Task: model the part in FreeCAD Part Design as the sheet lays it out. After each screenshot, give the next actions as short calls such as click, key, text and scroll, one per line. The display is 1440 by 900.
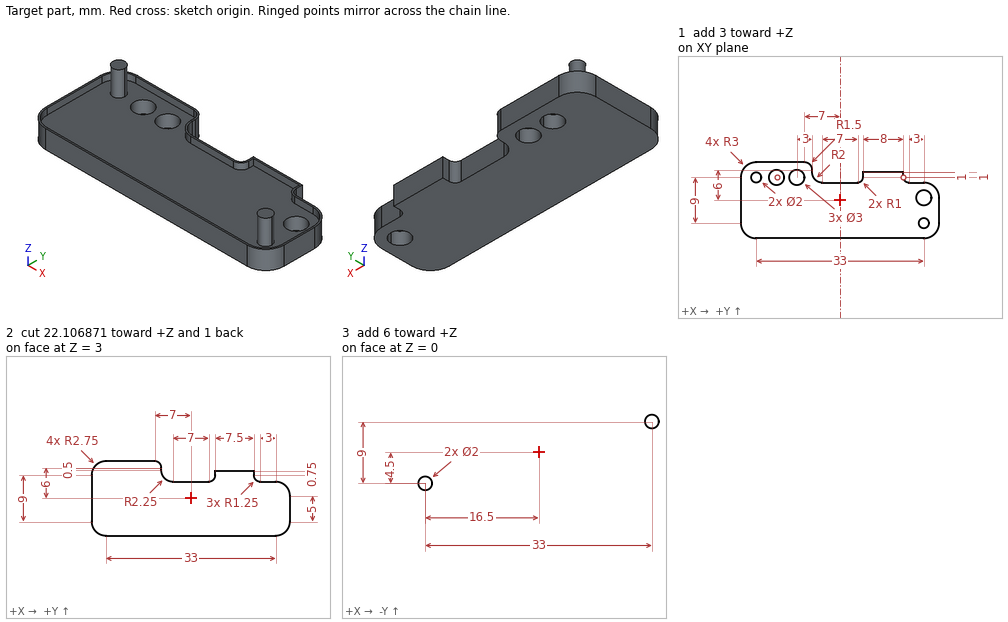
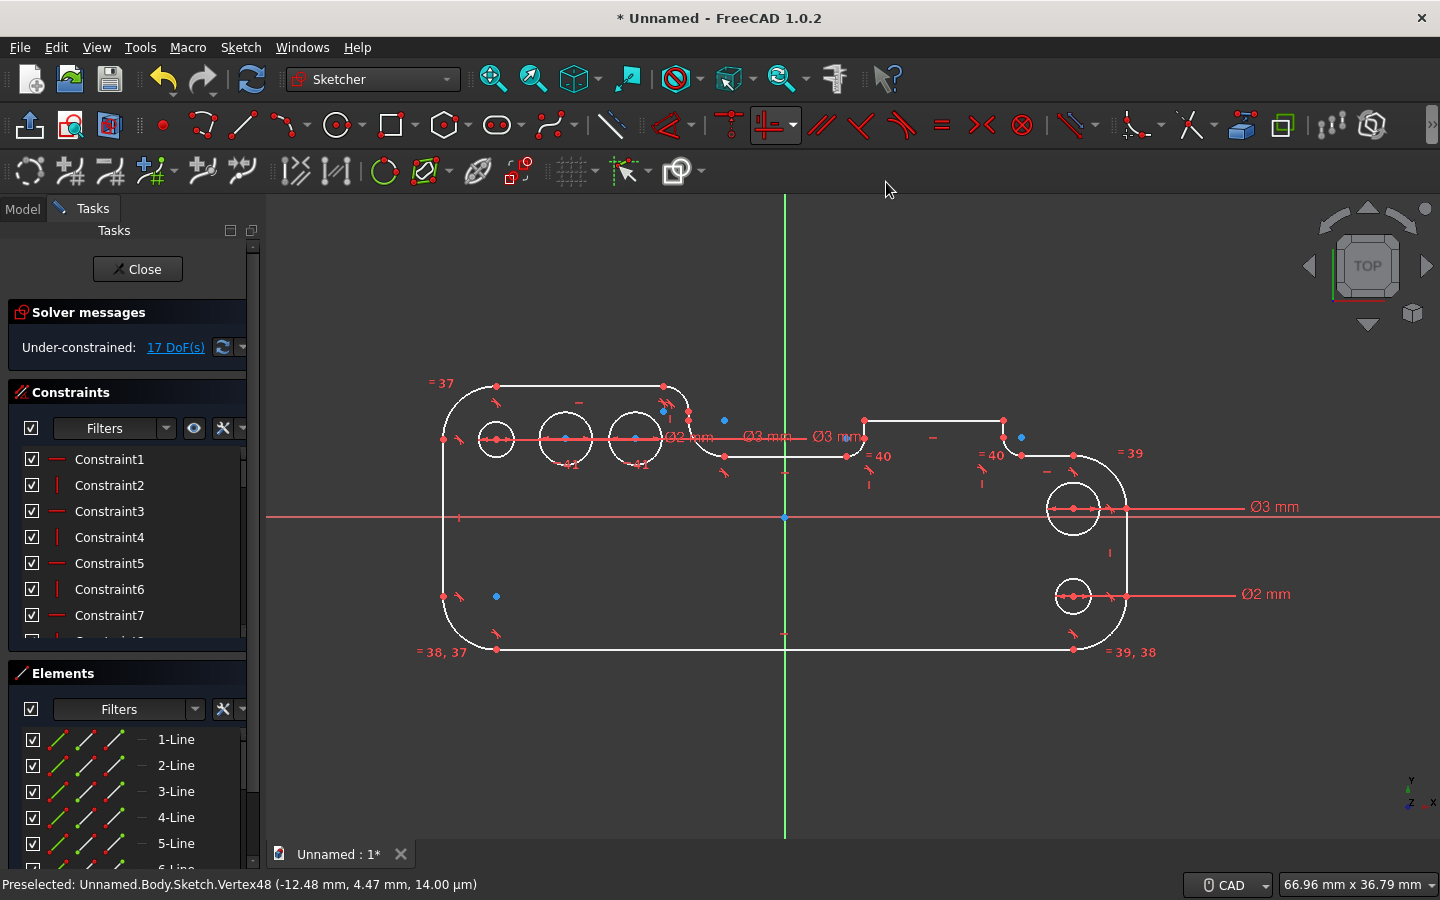
click(566, 439)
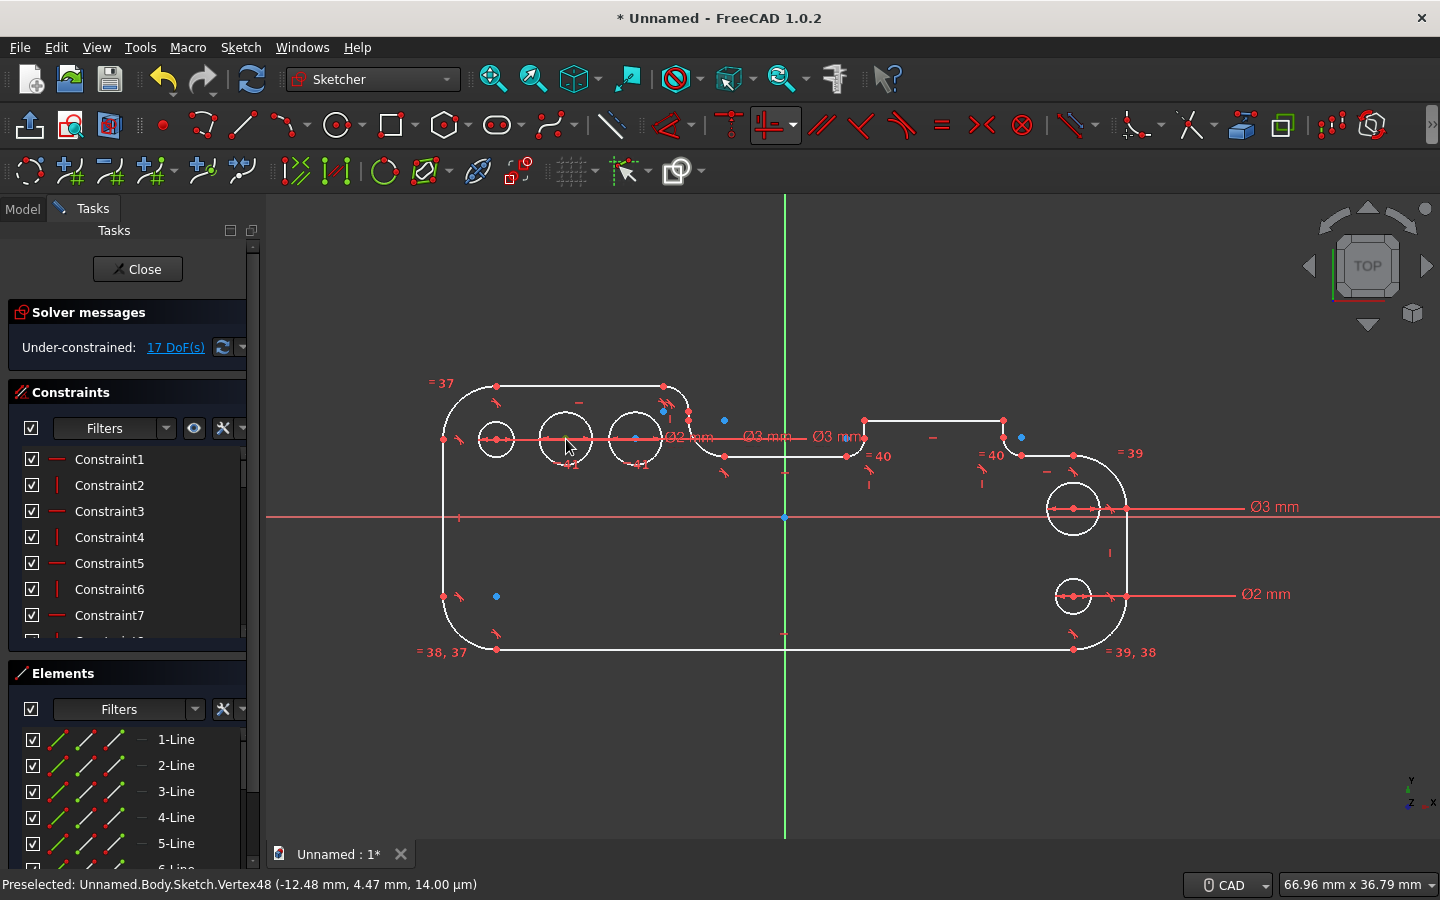
click(496, 440)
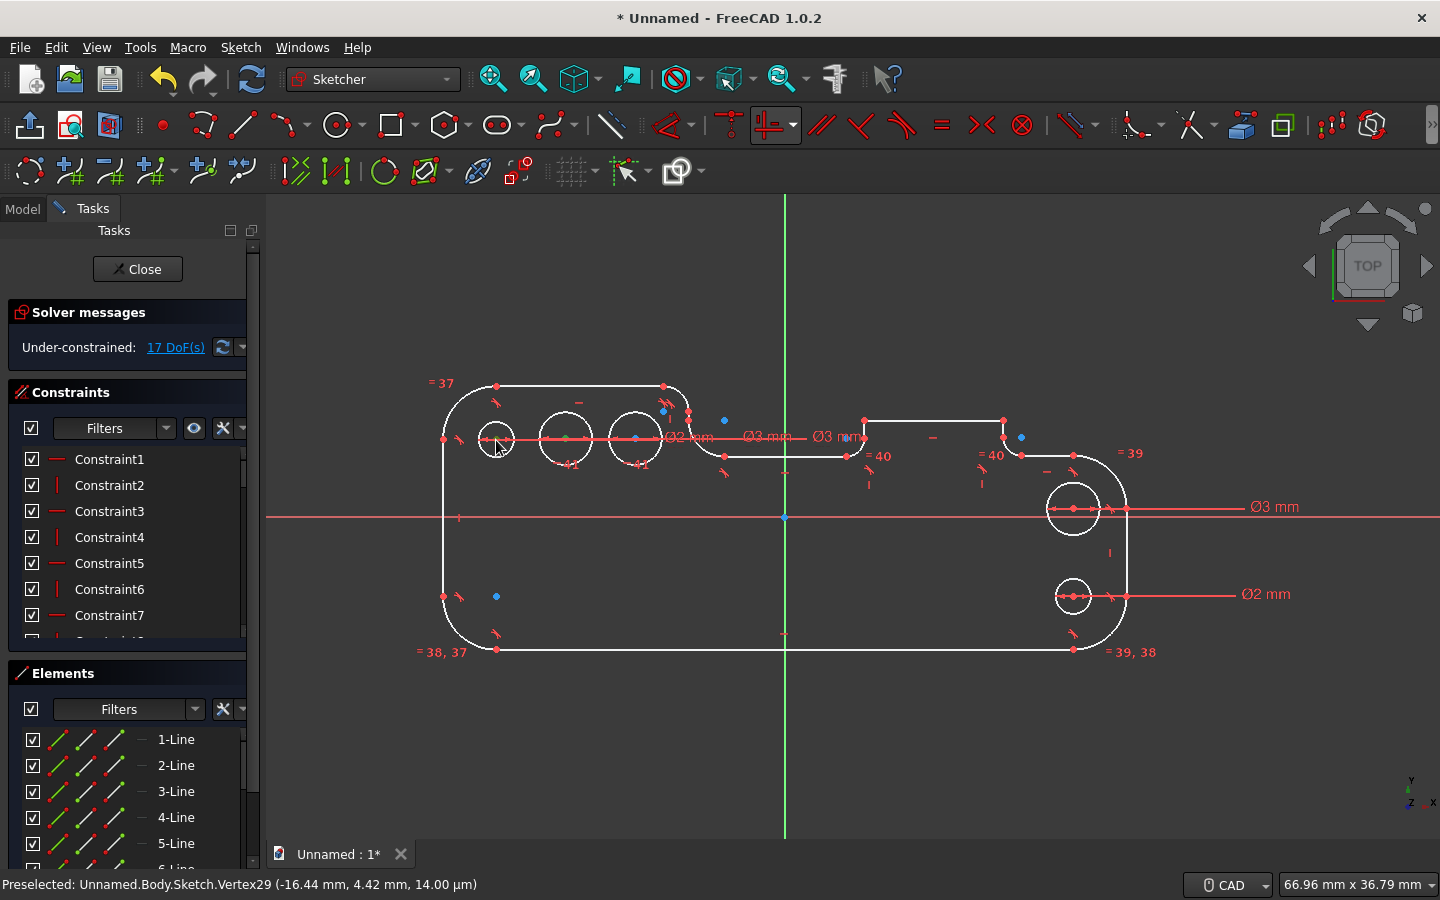
click(796, 126)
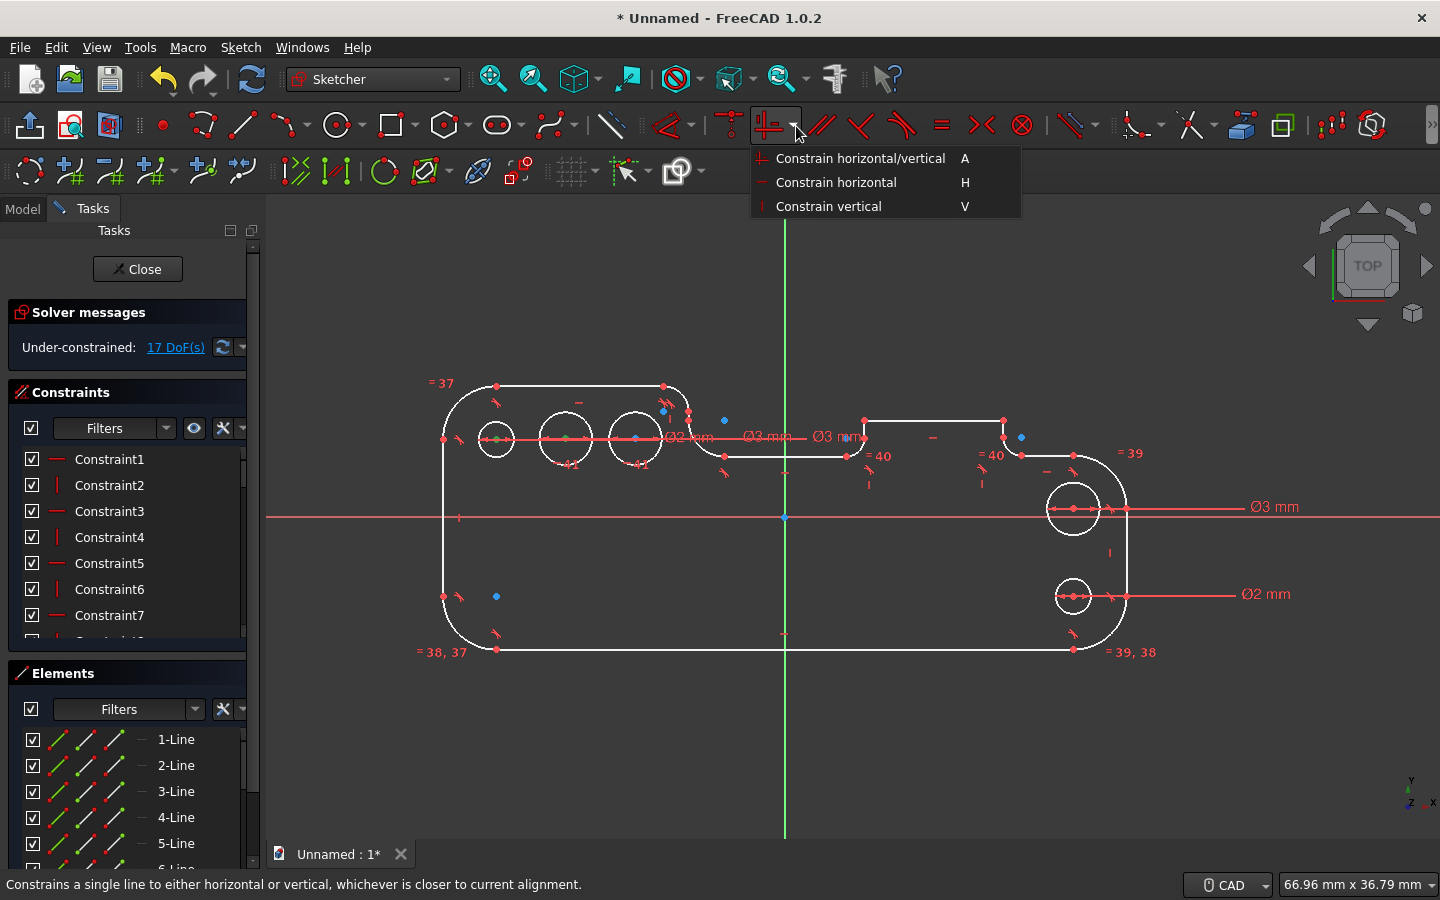
click(886, 182)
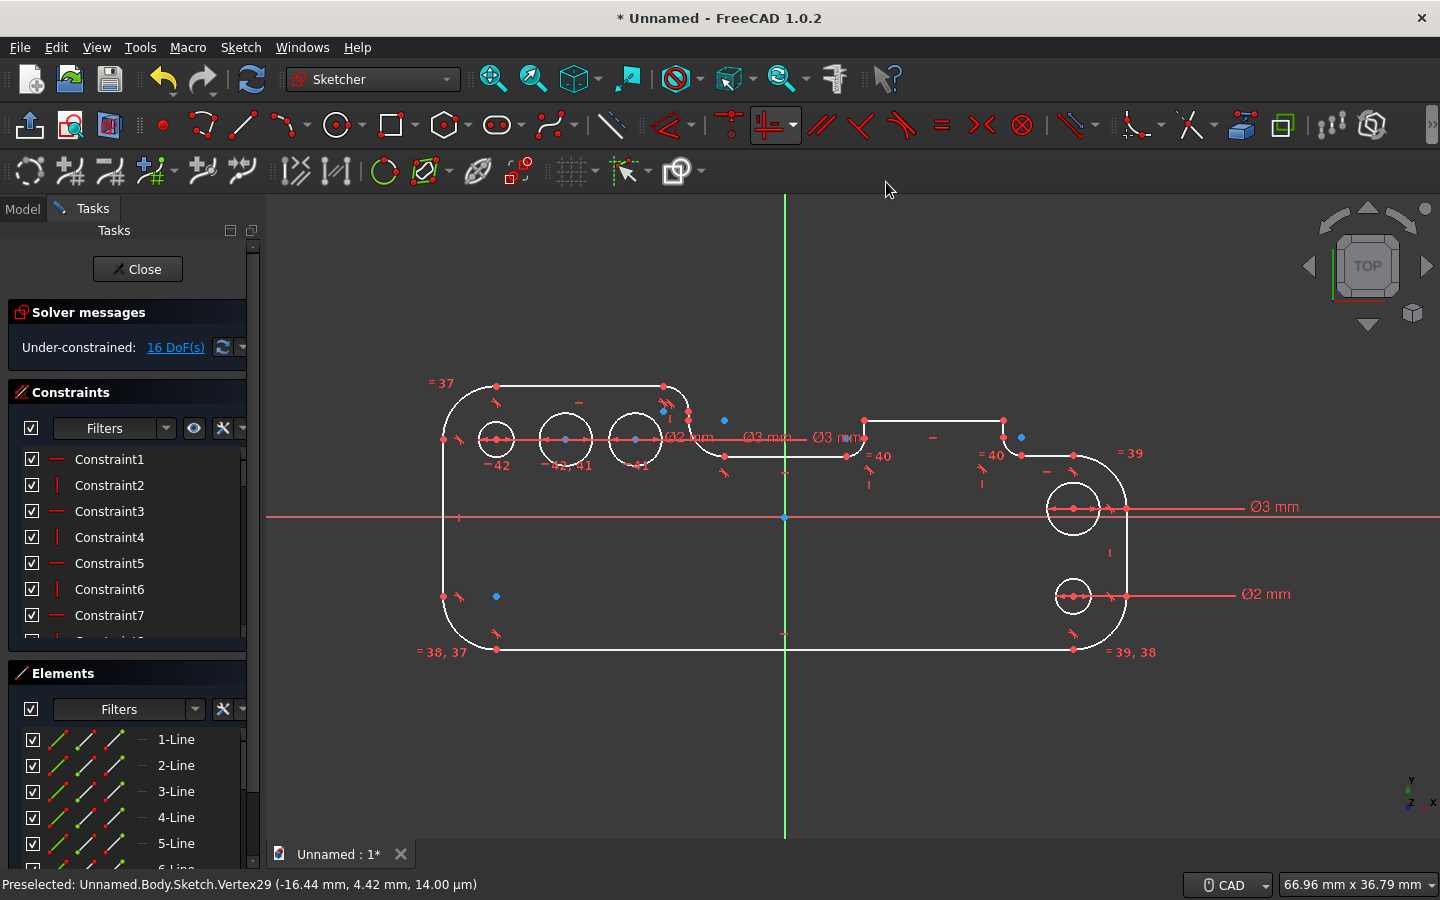
click(566, 440)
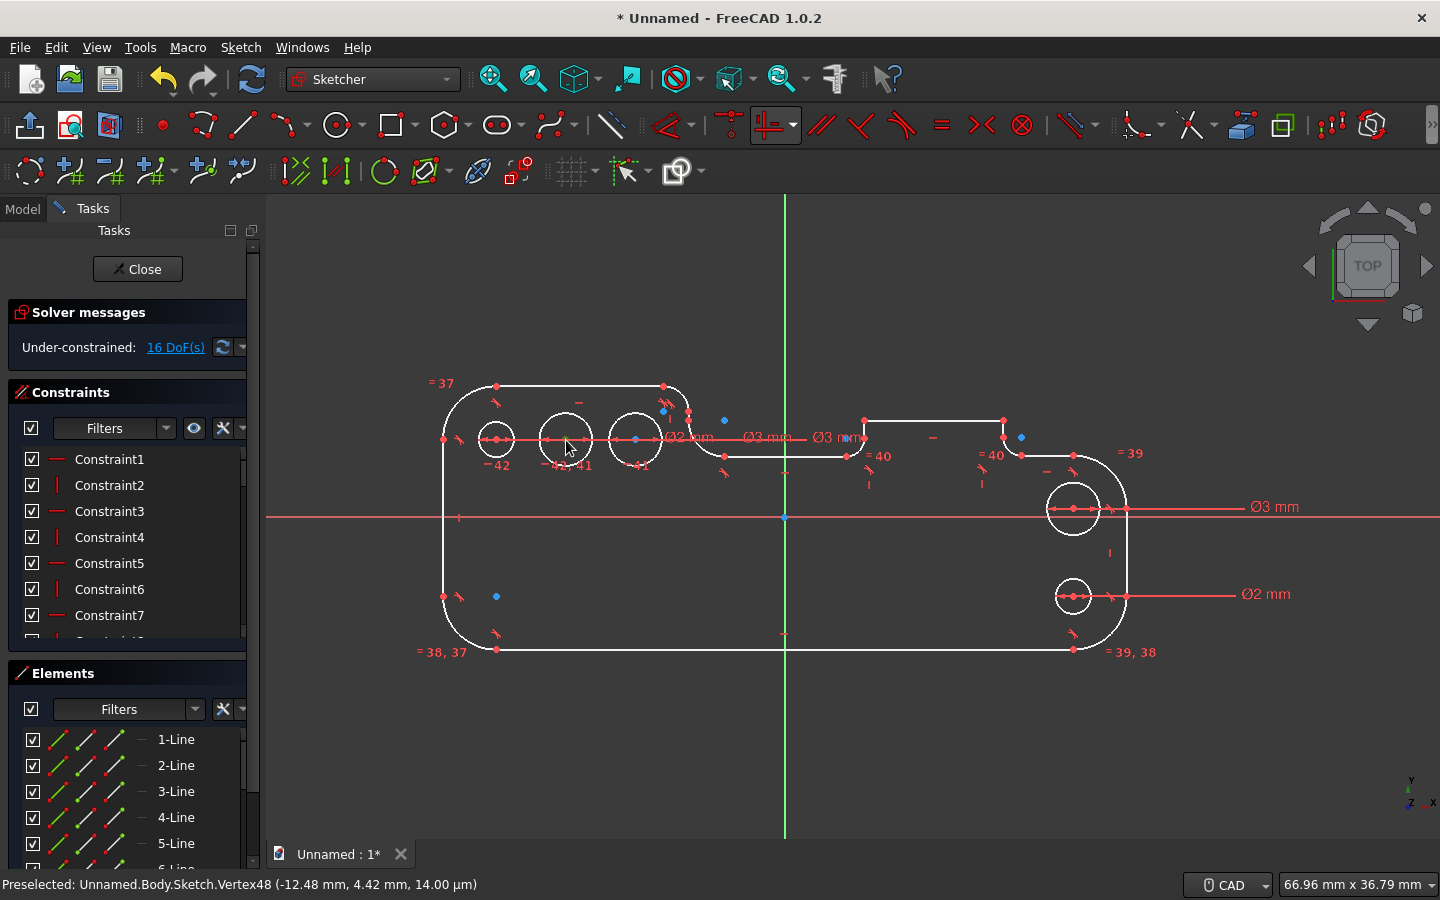
click(1003, 438)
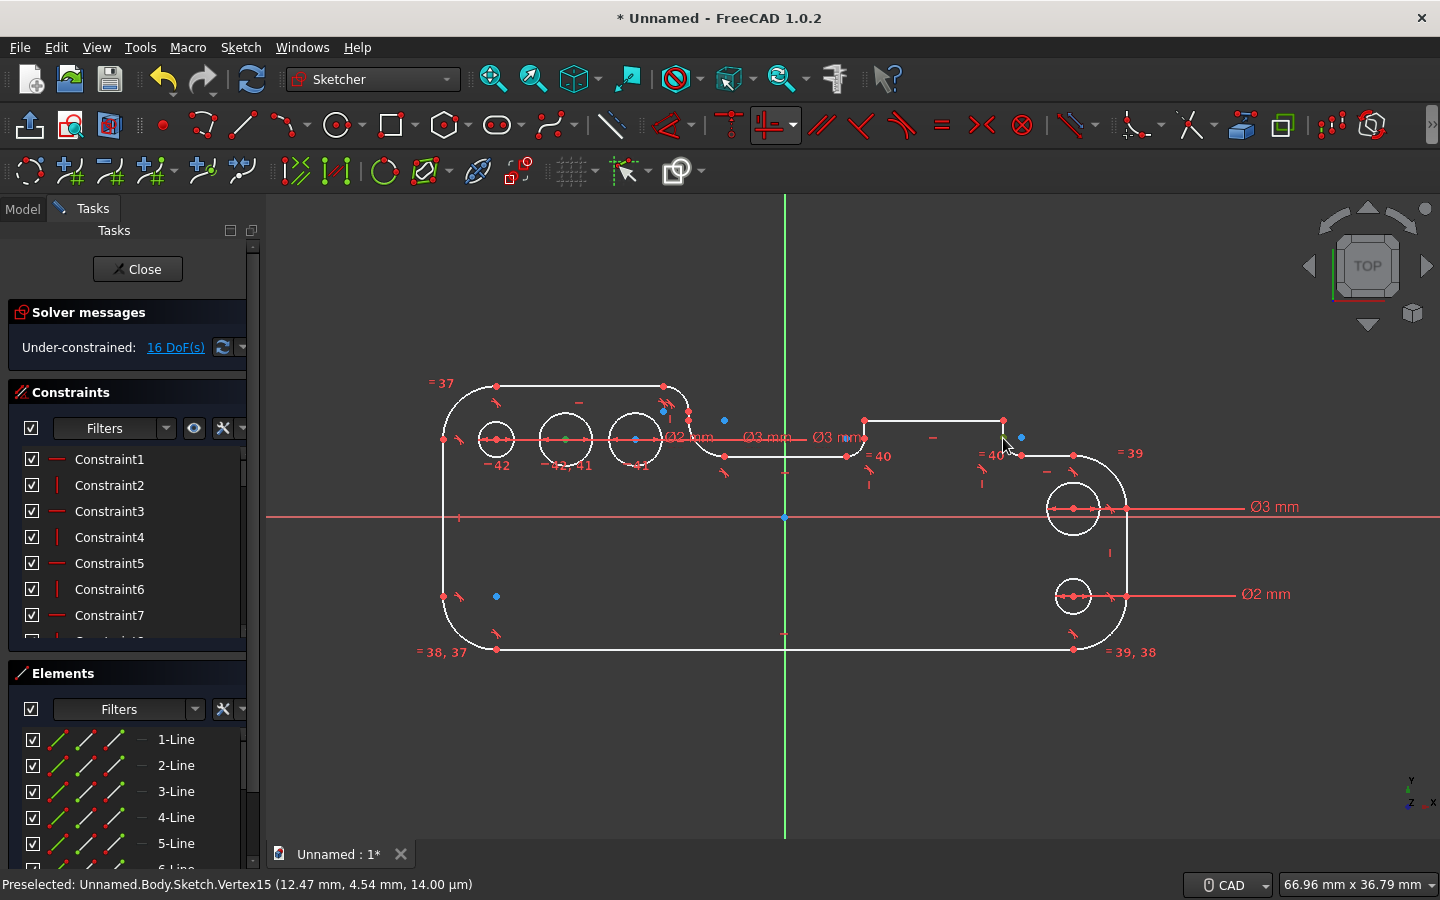
click(785, 769)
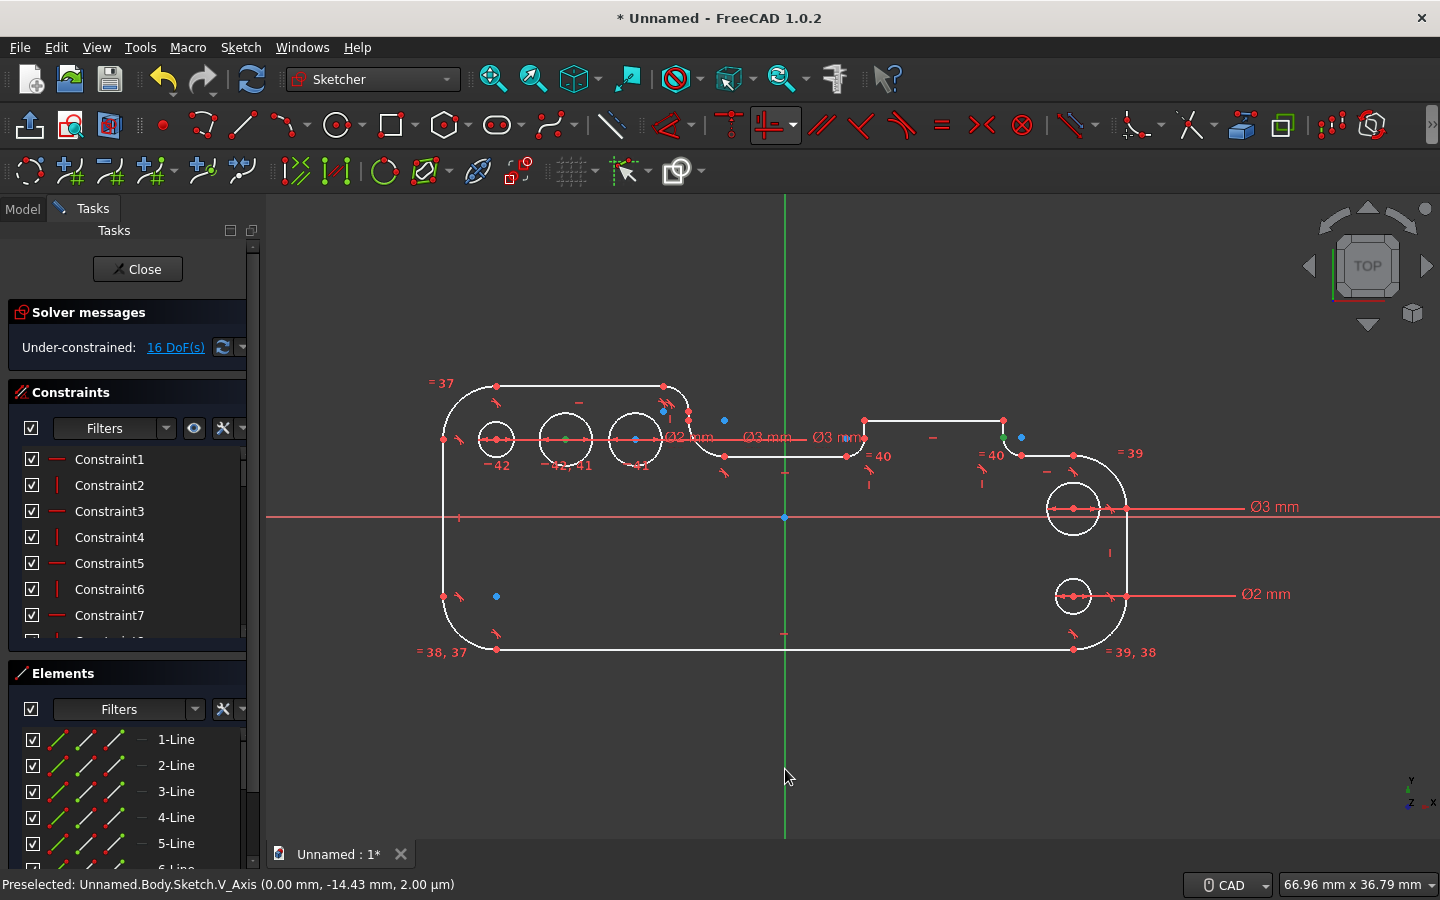
click(982, 126)